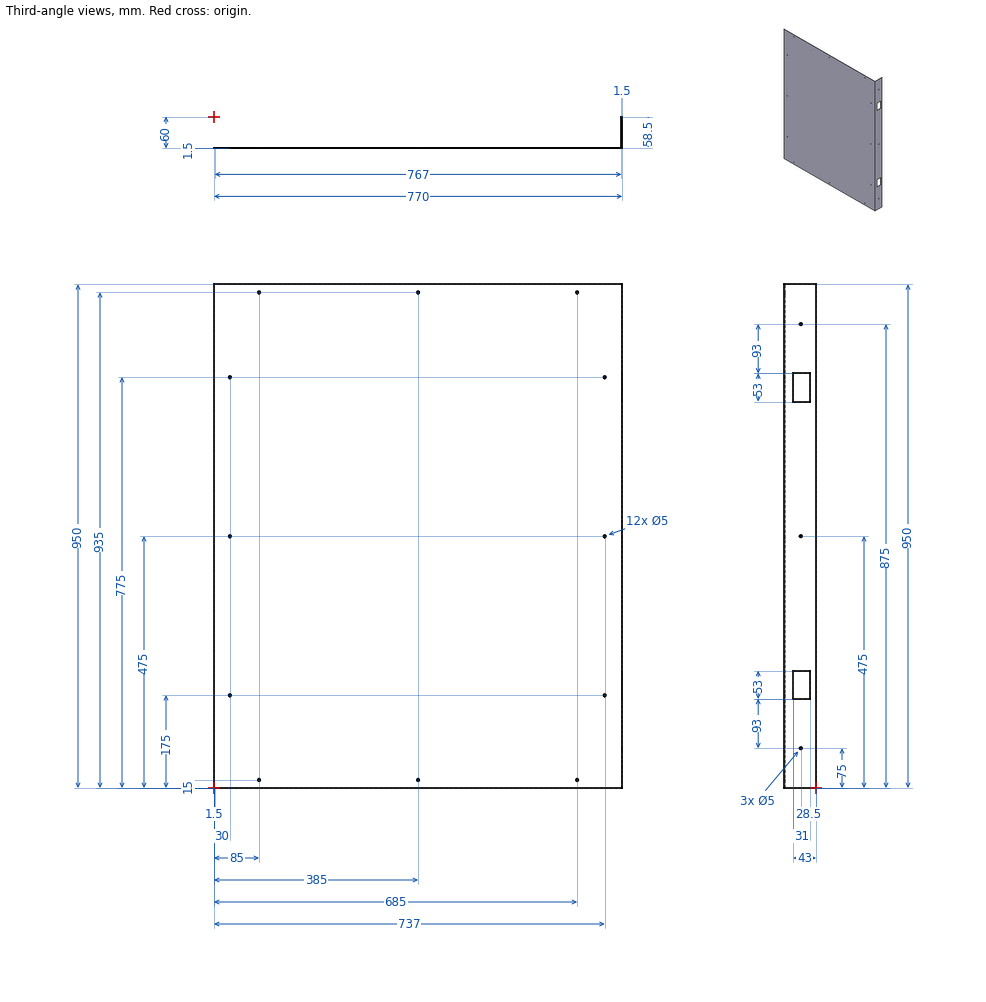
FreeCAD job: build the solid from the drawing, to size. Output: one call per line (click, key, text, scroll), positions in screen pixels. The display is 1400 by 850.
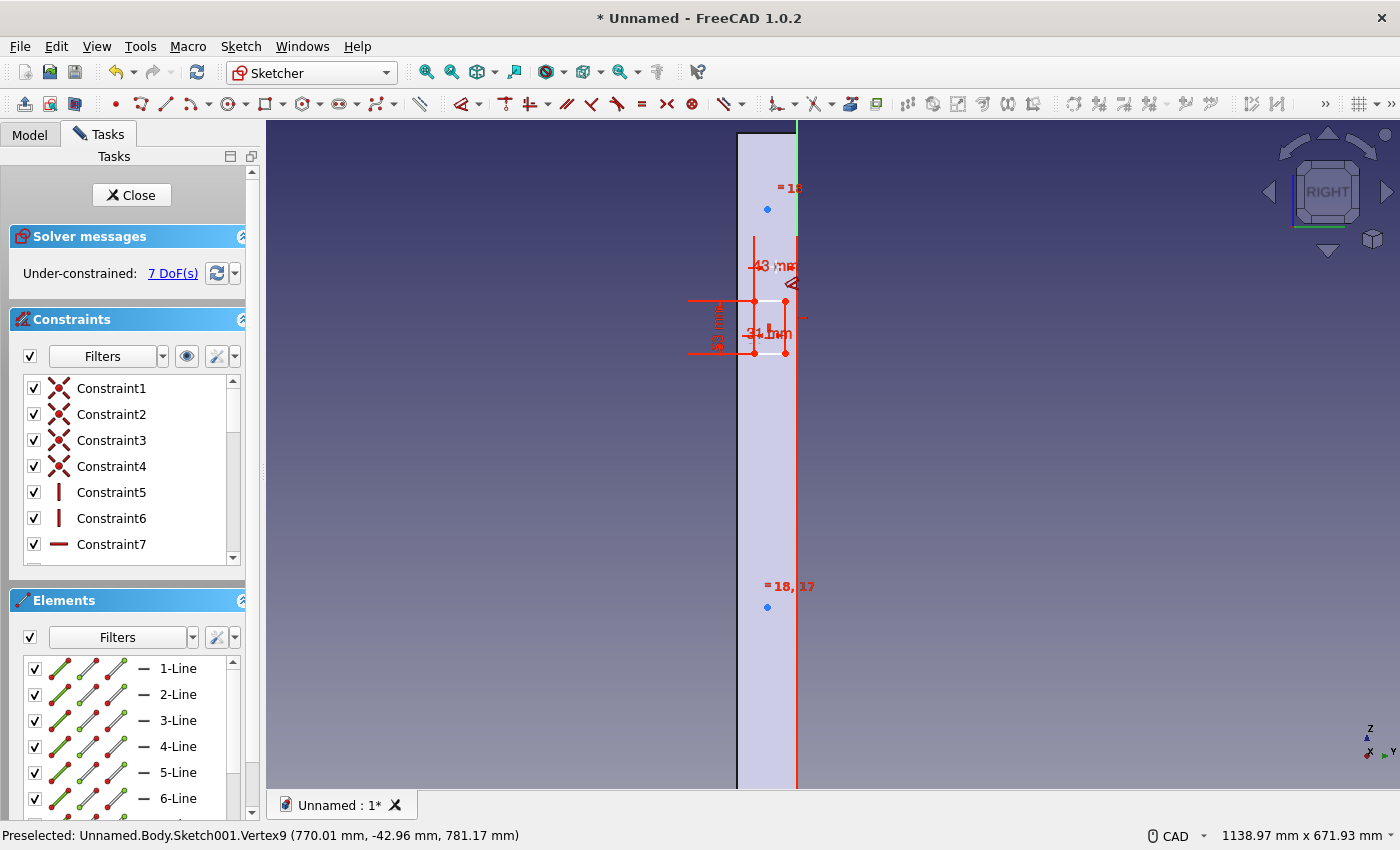
click(768, 607)
click(831, 684)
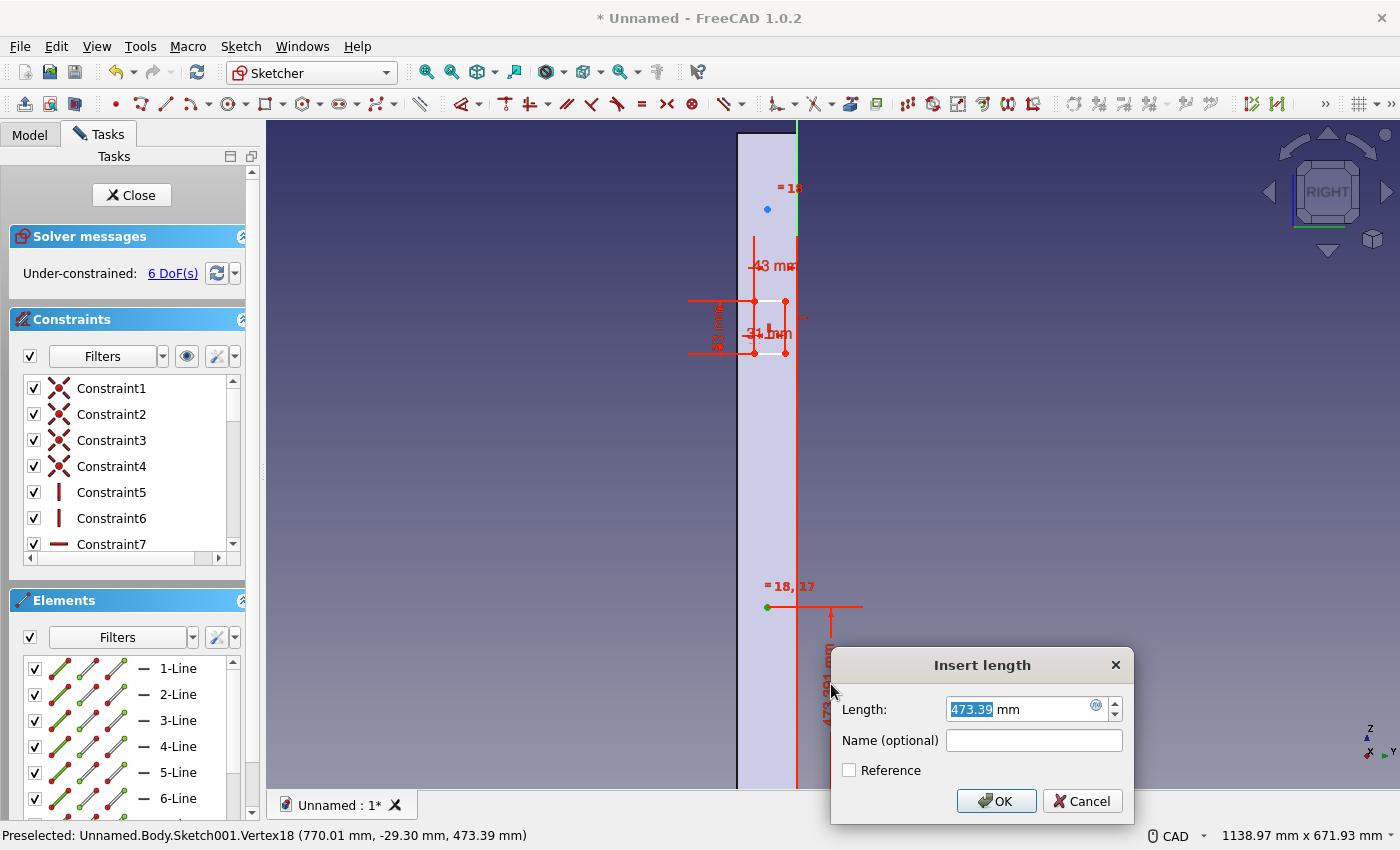
text(475)
key(Return)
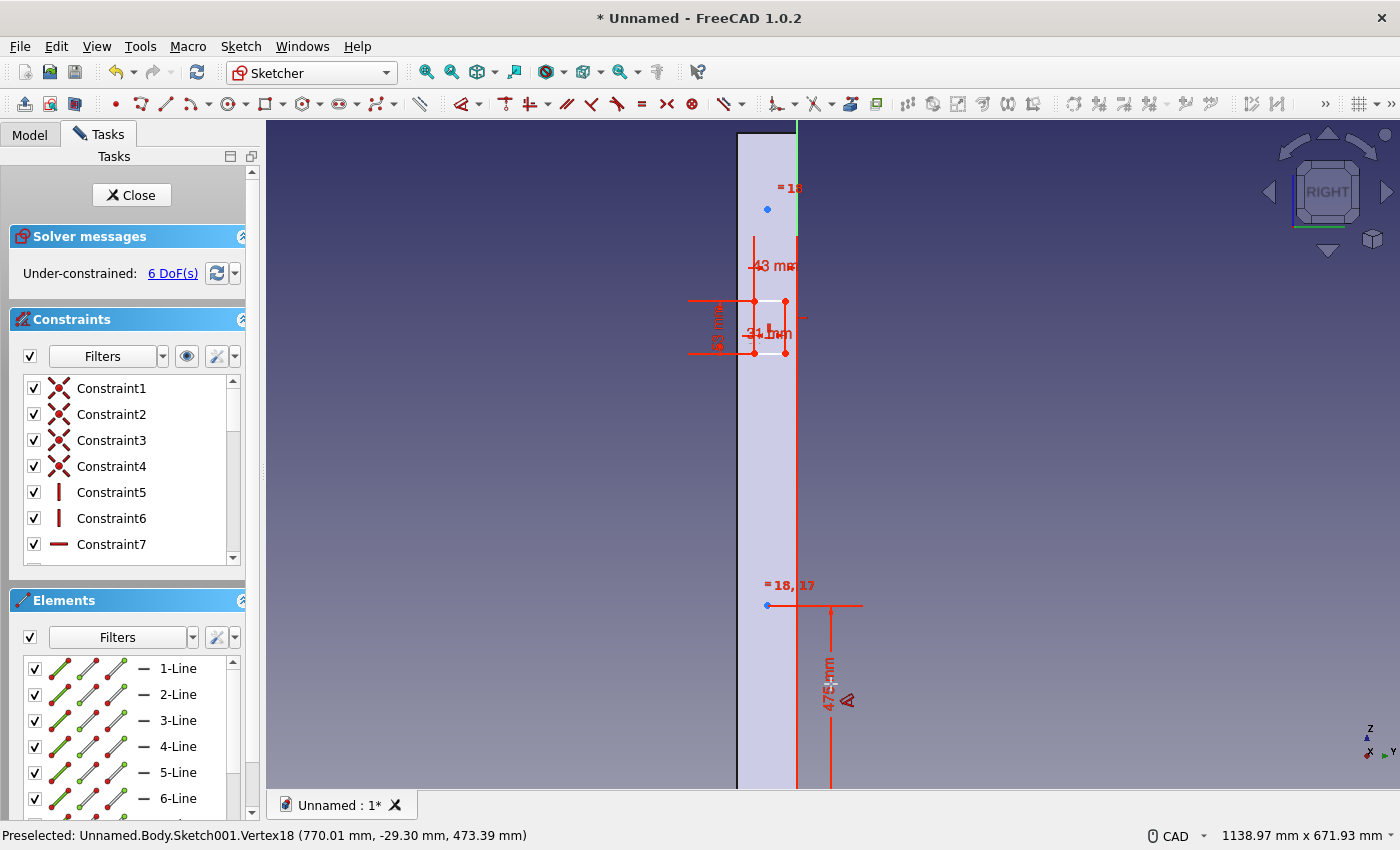
click(768, 210)
click(831, 485)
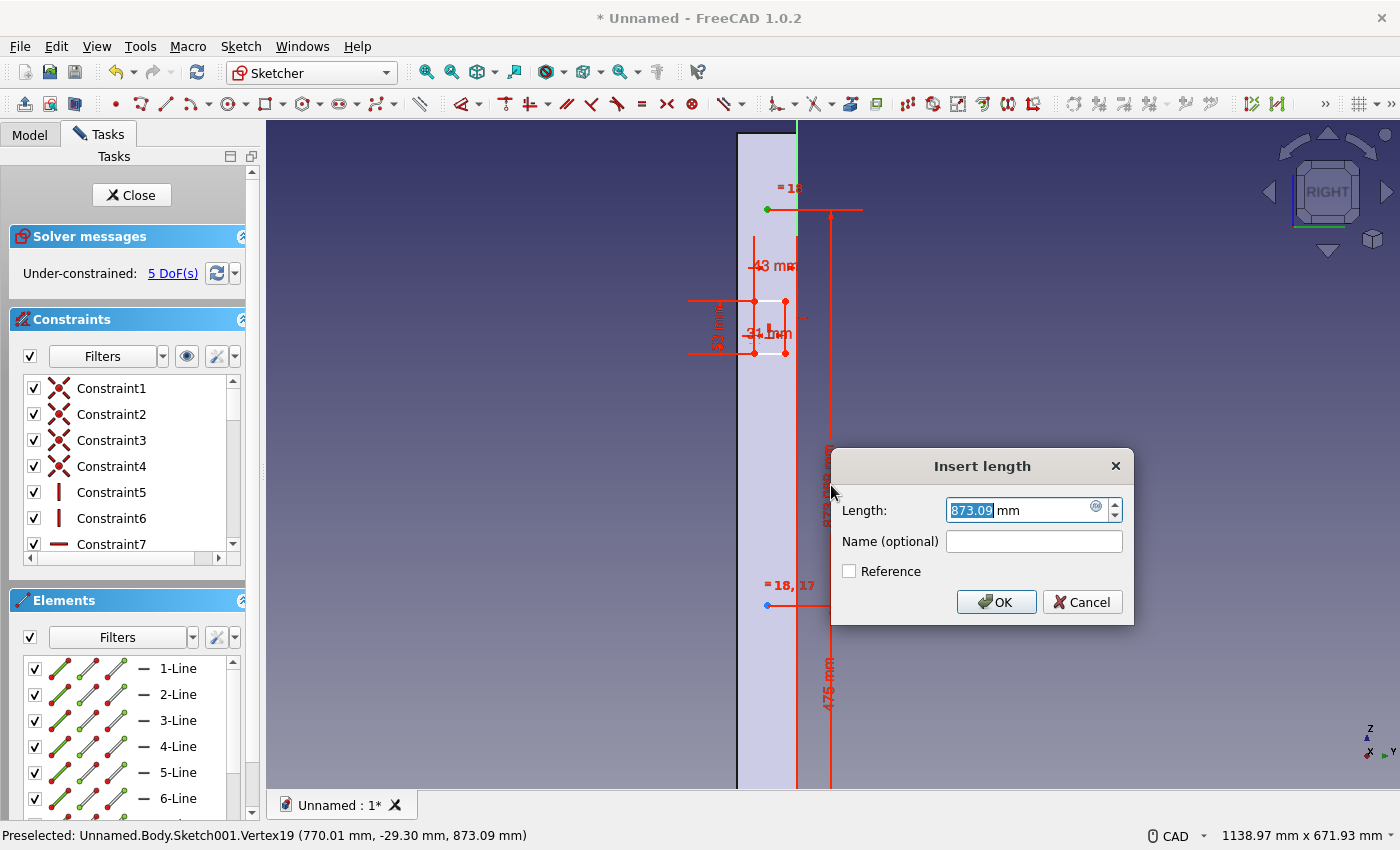
text(875)
key(Return)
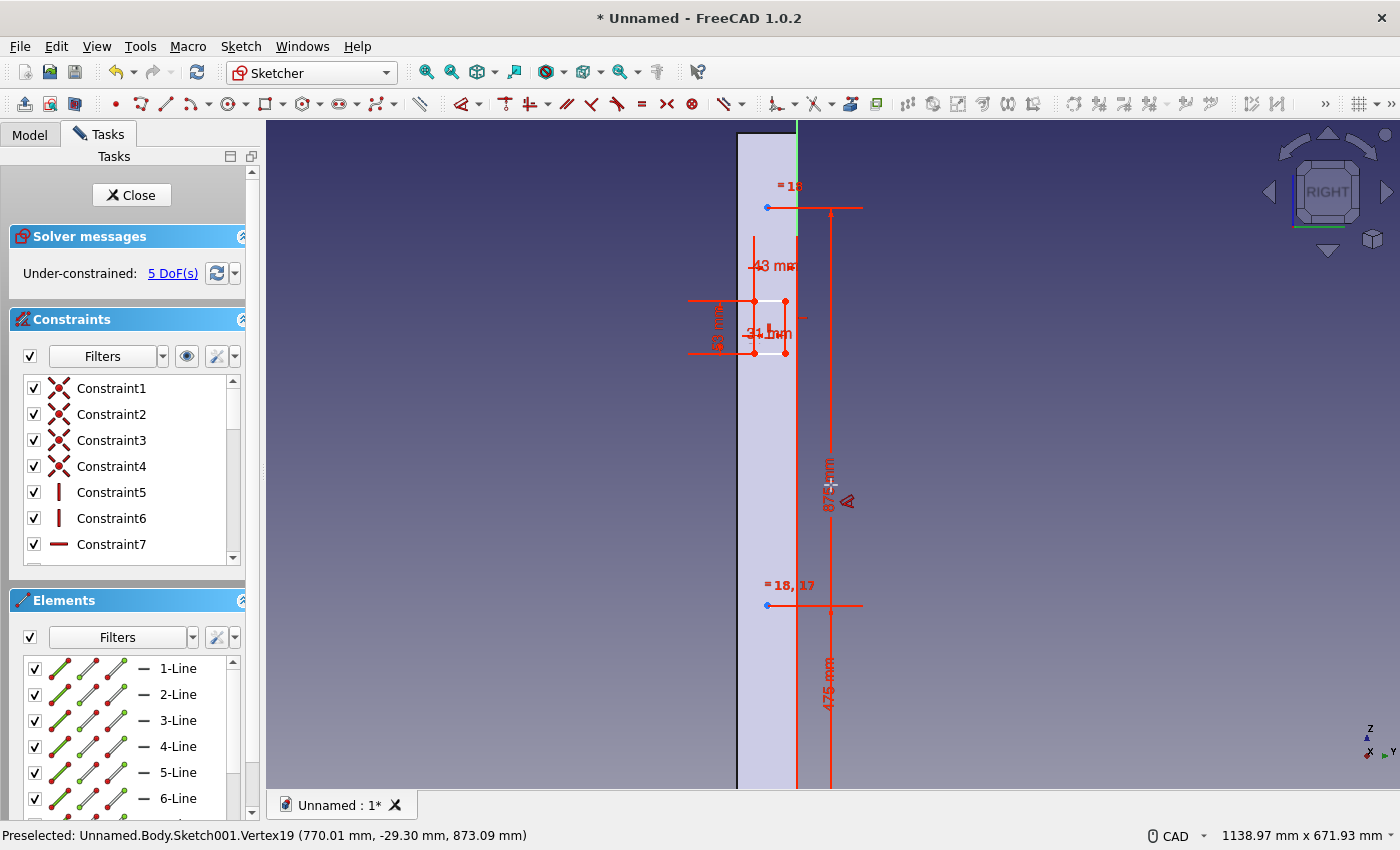
scroll(755, 302, down, 4)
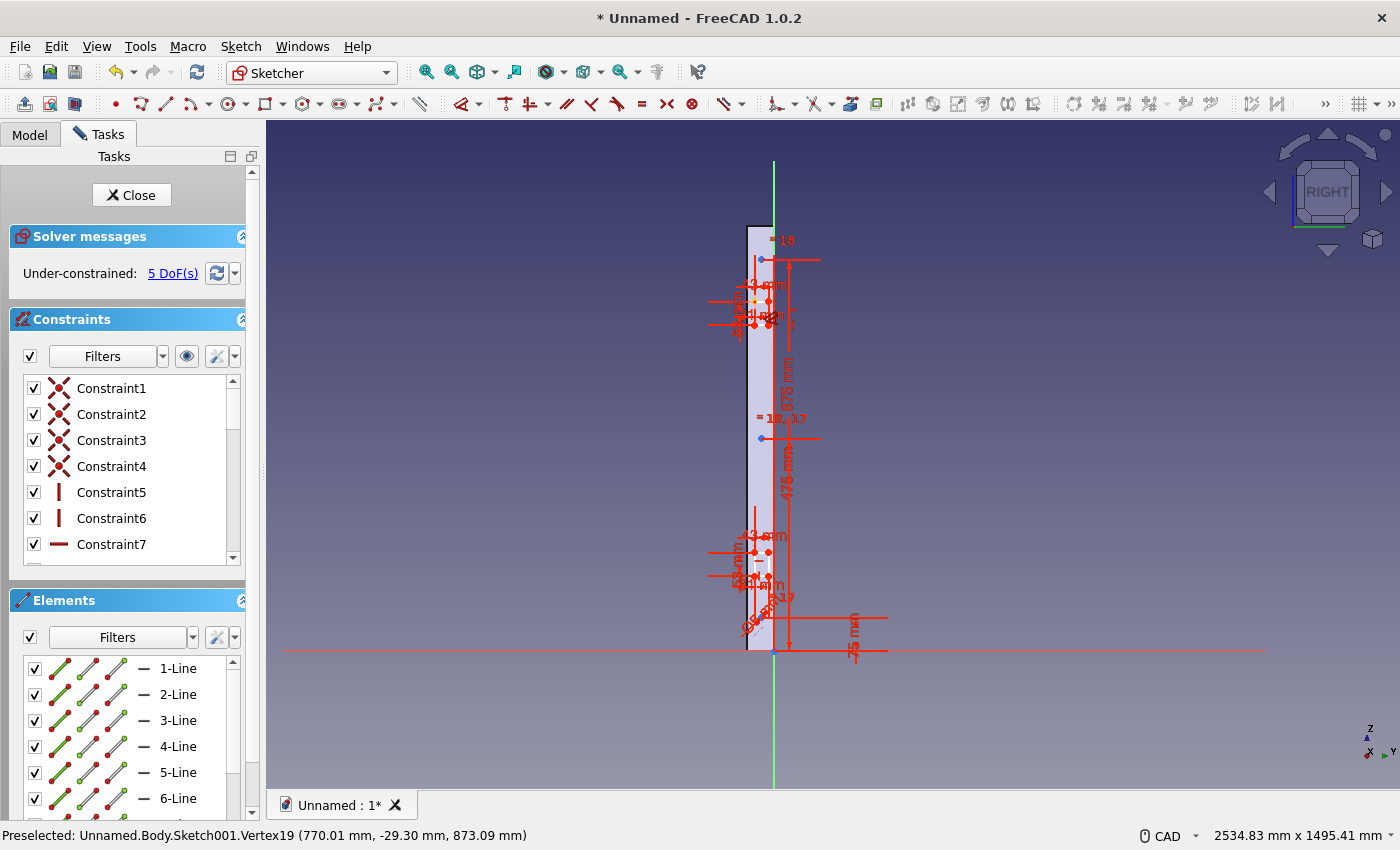
click(755, 576)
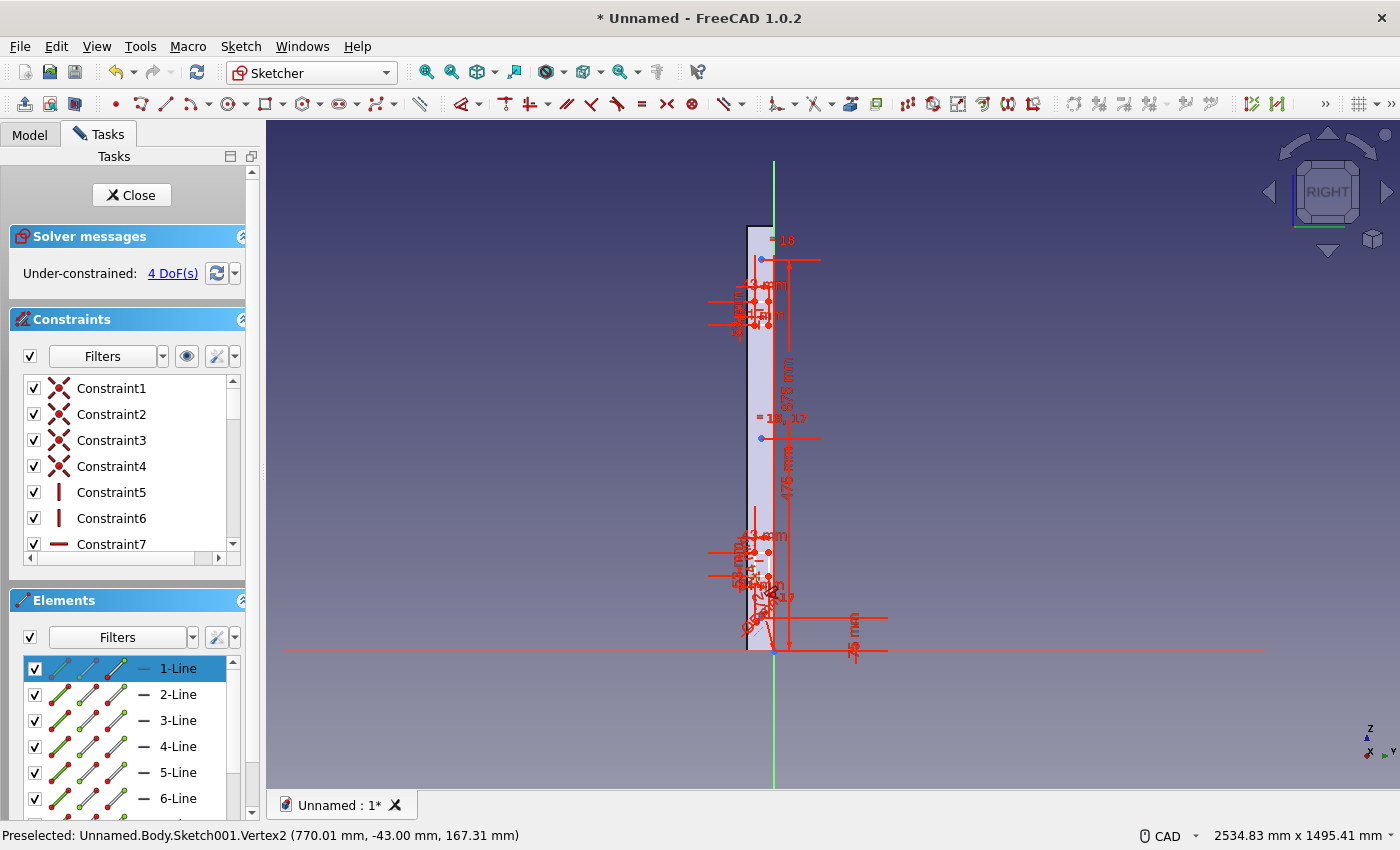
click(761, 618)
click(673, 597)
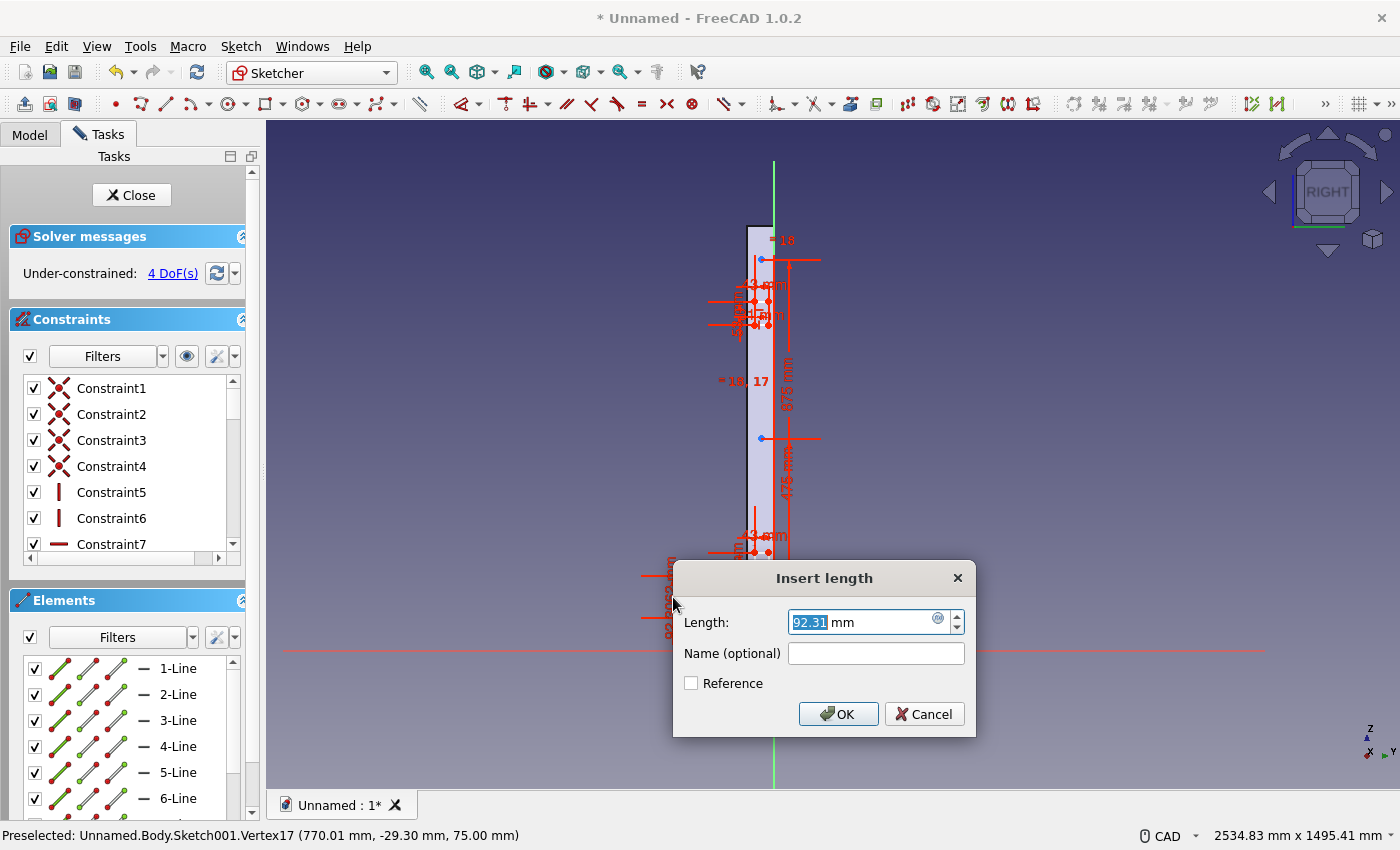
text(93)
key(Return)